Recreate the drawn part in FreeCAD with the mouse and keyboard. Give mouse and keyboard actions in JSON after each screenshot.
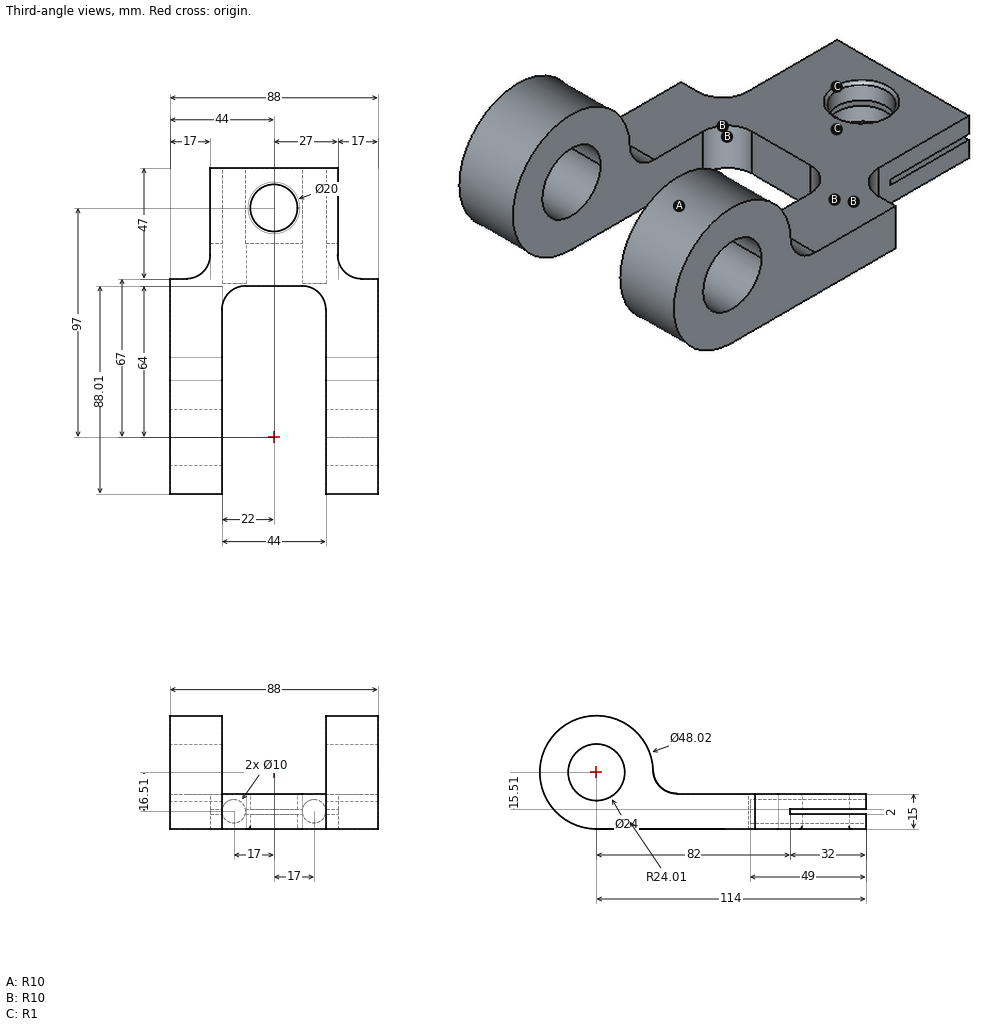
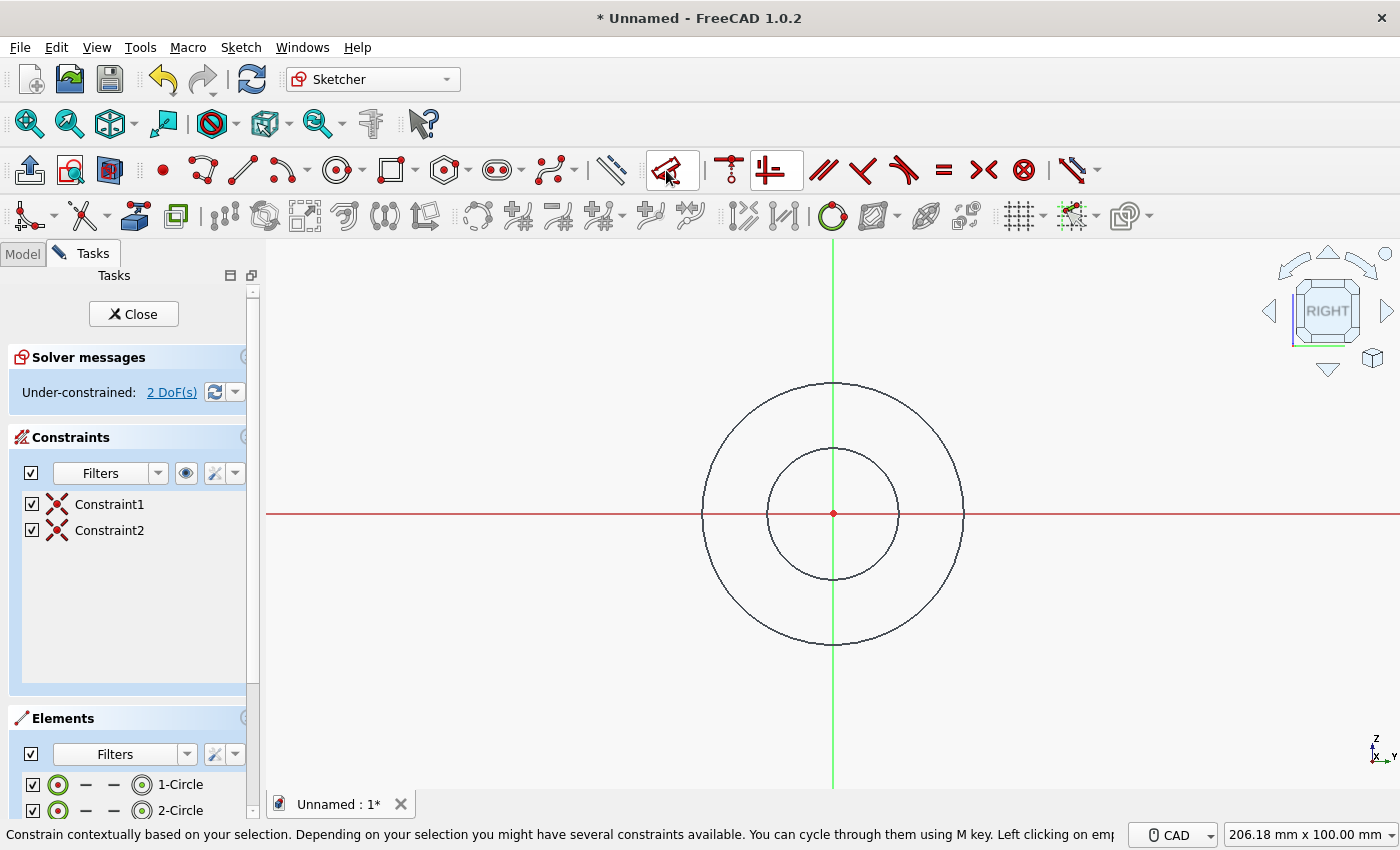
{"action": "left_click", "coordinate": [925, 421]}
{"action": "left_click", "coordinate": [948, 398]}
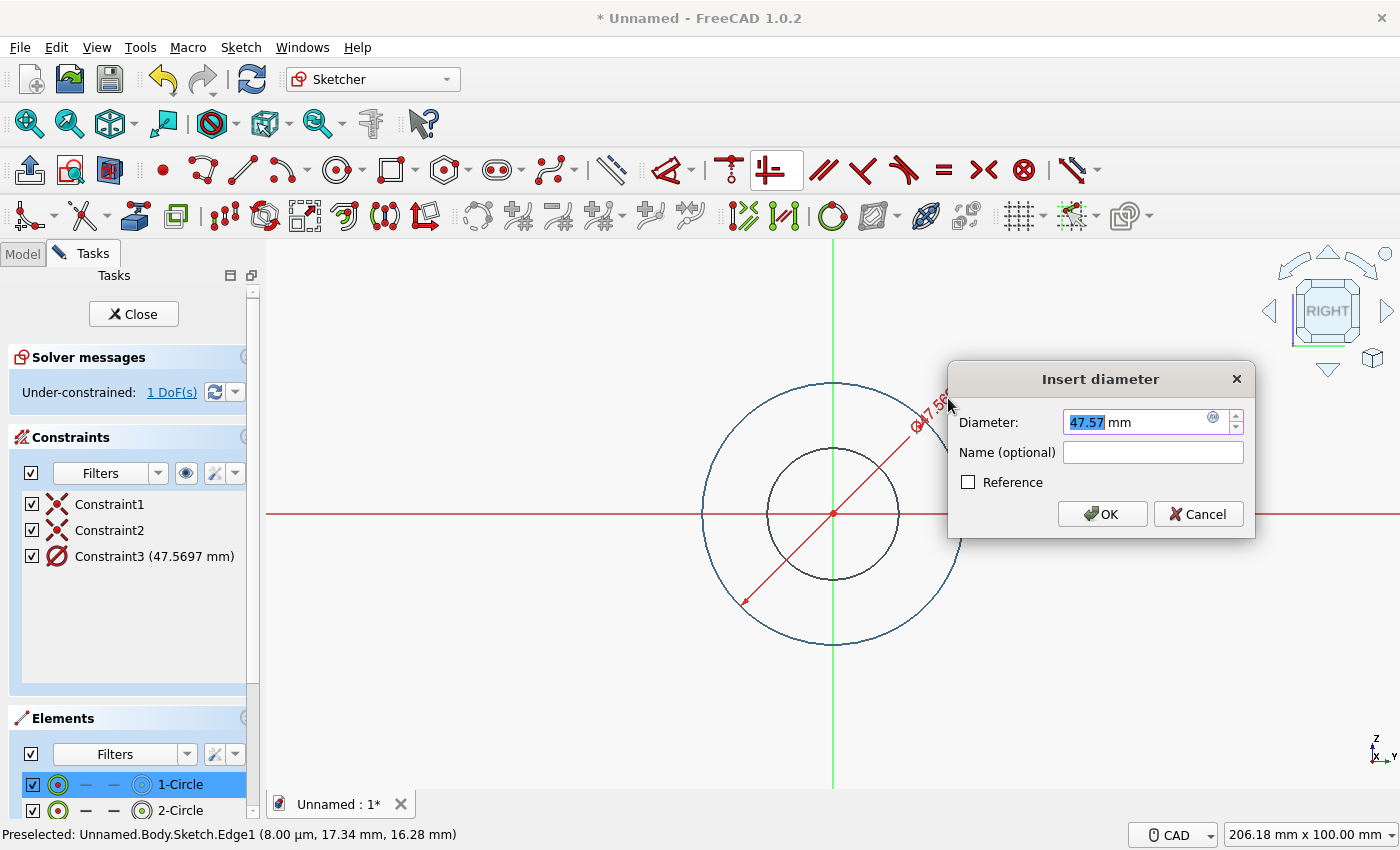
{"action": "type", "text": "48.02"}
{"action": "key", "text": "Return"}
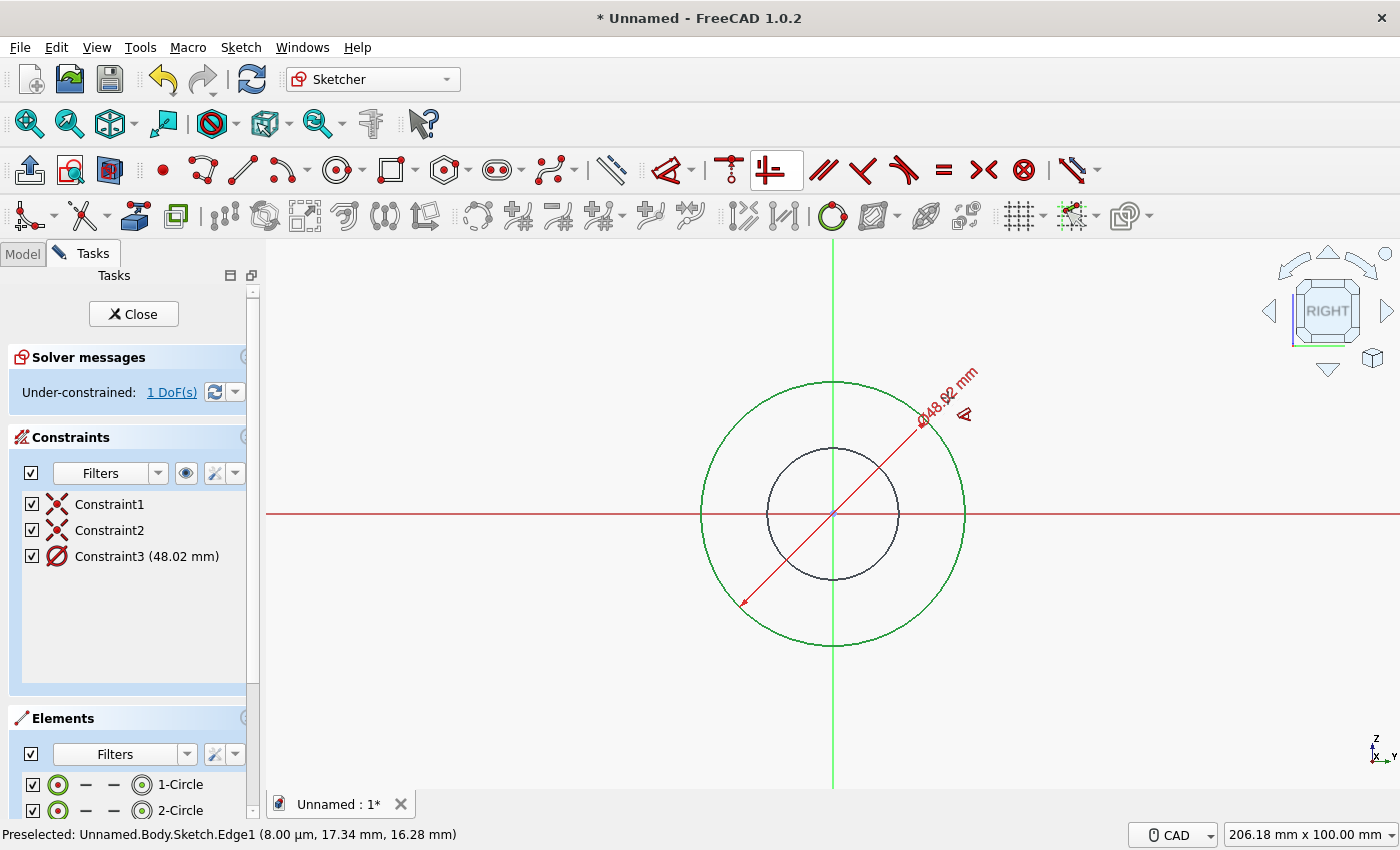
{"action": "left_click", "coordinate": [879, 467]}
{"action": "left_click", "coordinate": [901, 444]}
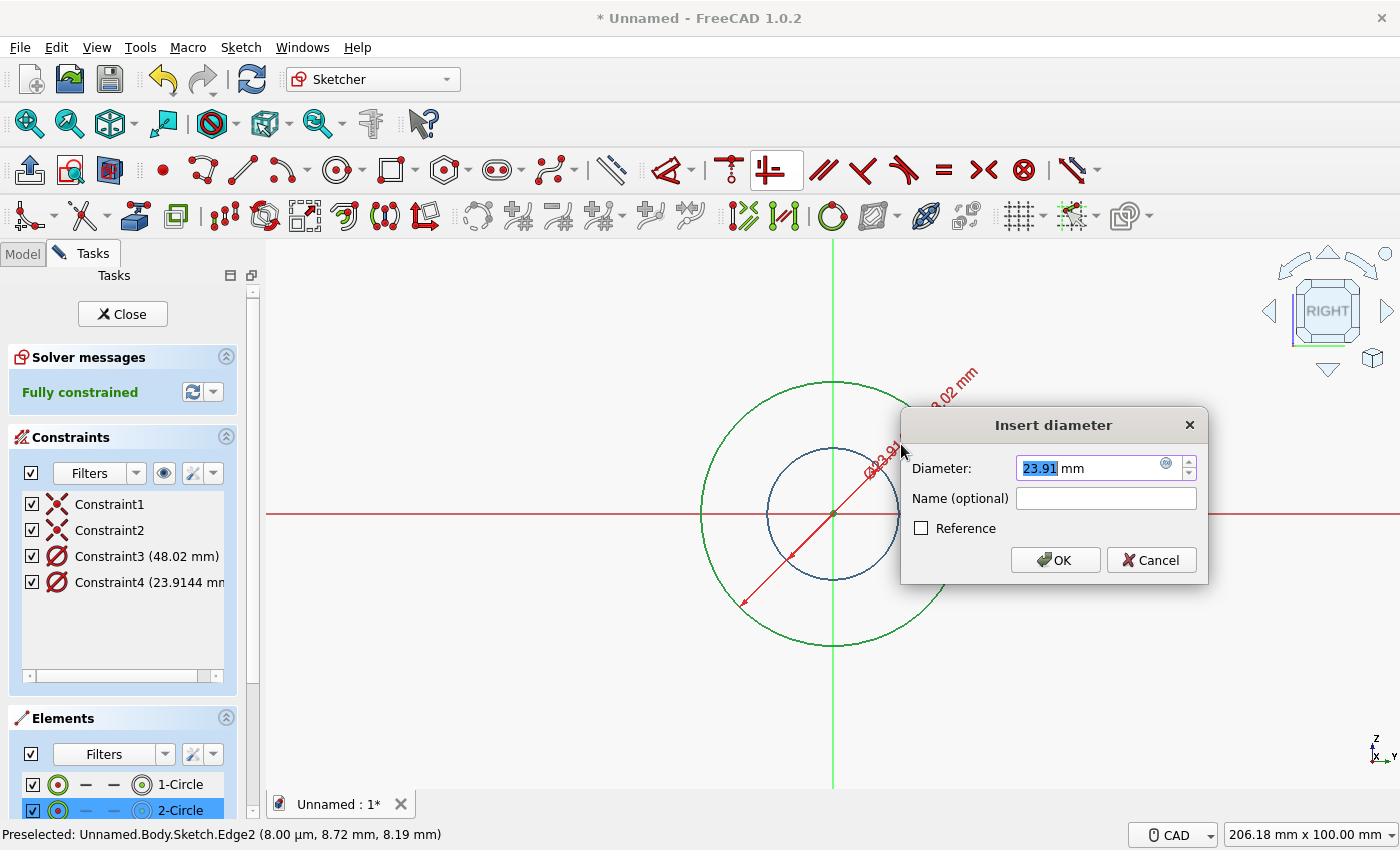
{"action": "type", "text": "24"}
{"action": "key", "text": "Return"}
{"action": "key", "text": "Escape"}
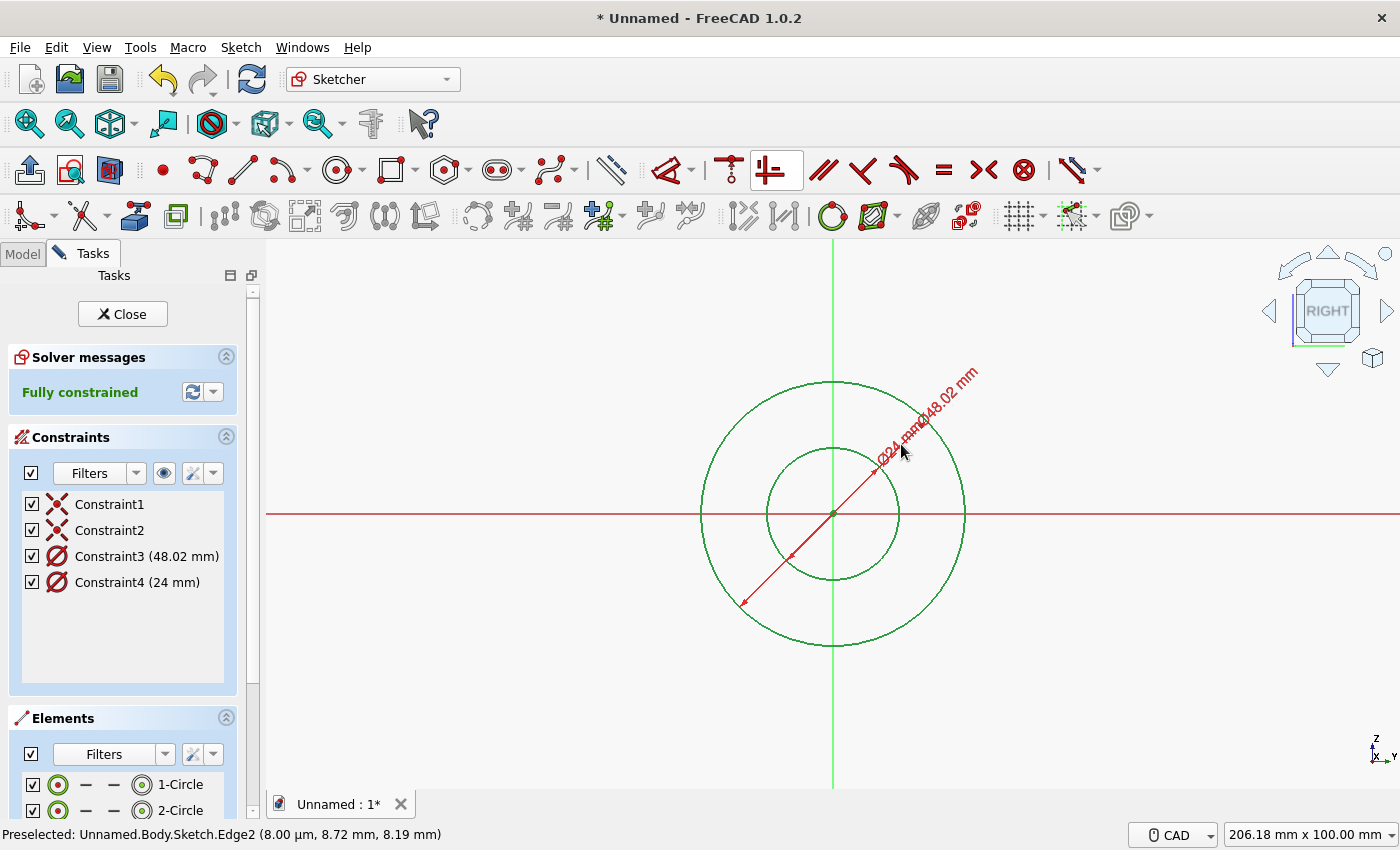
{"action": "left_click", "coordinate": [123, 314]}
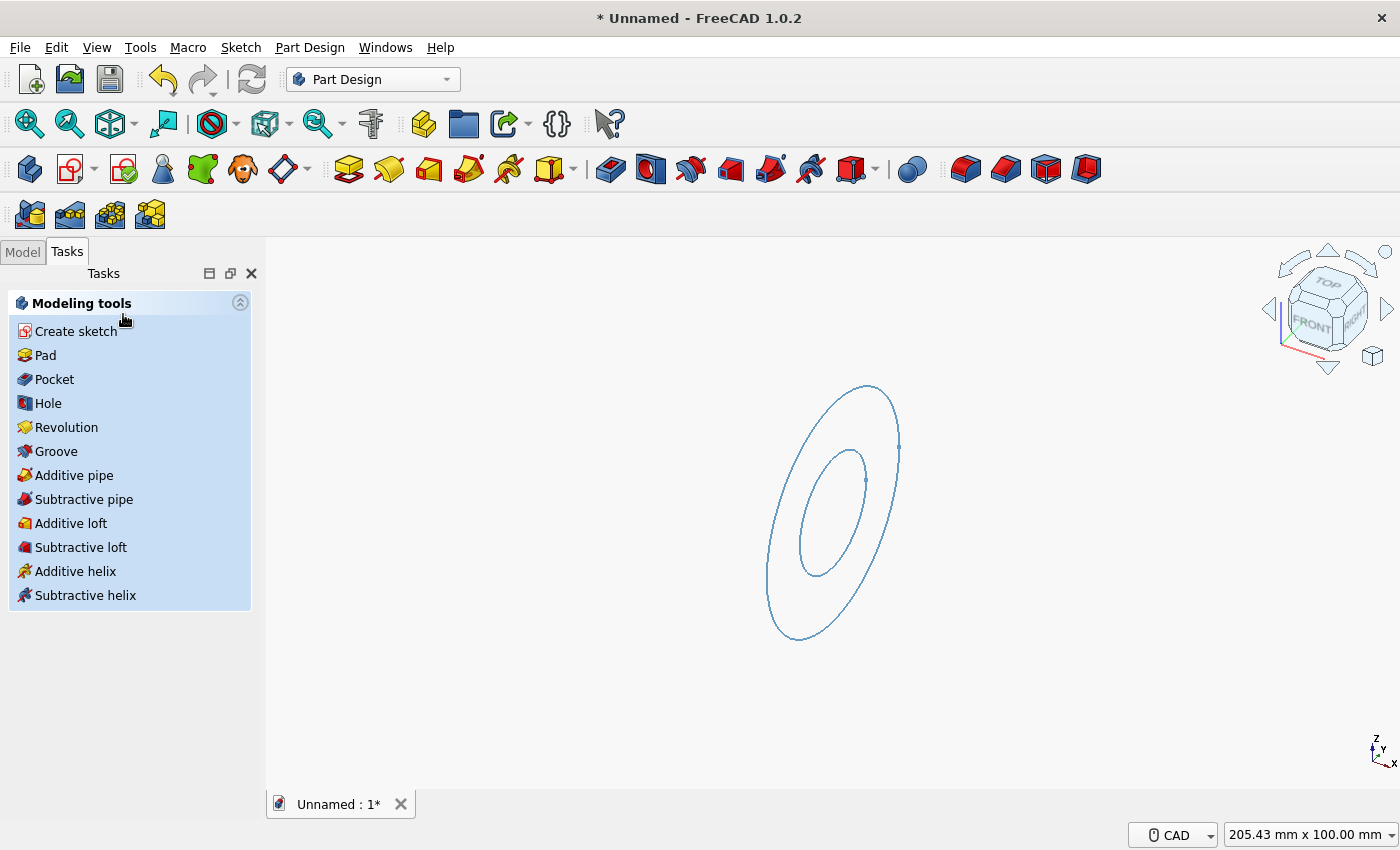
{"action": "left_click", "coordinate": [350, 170]}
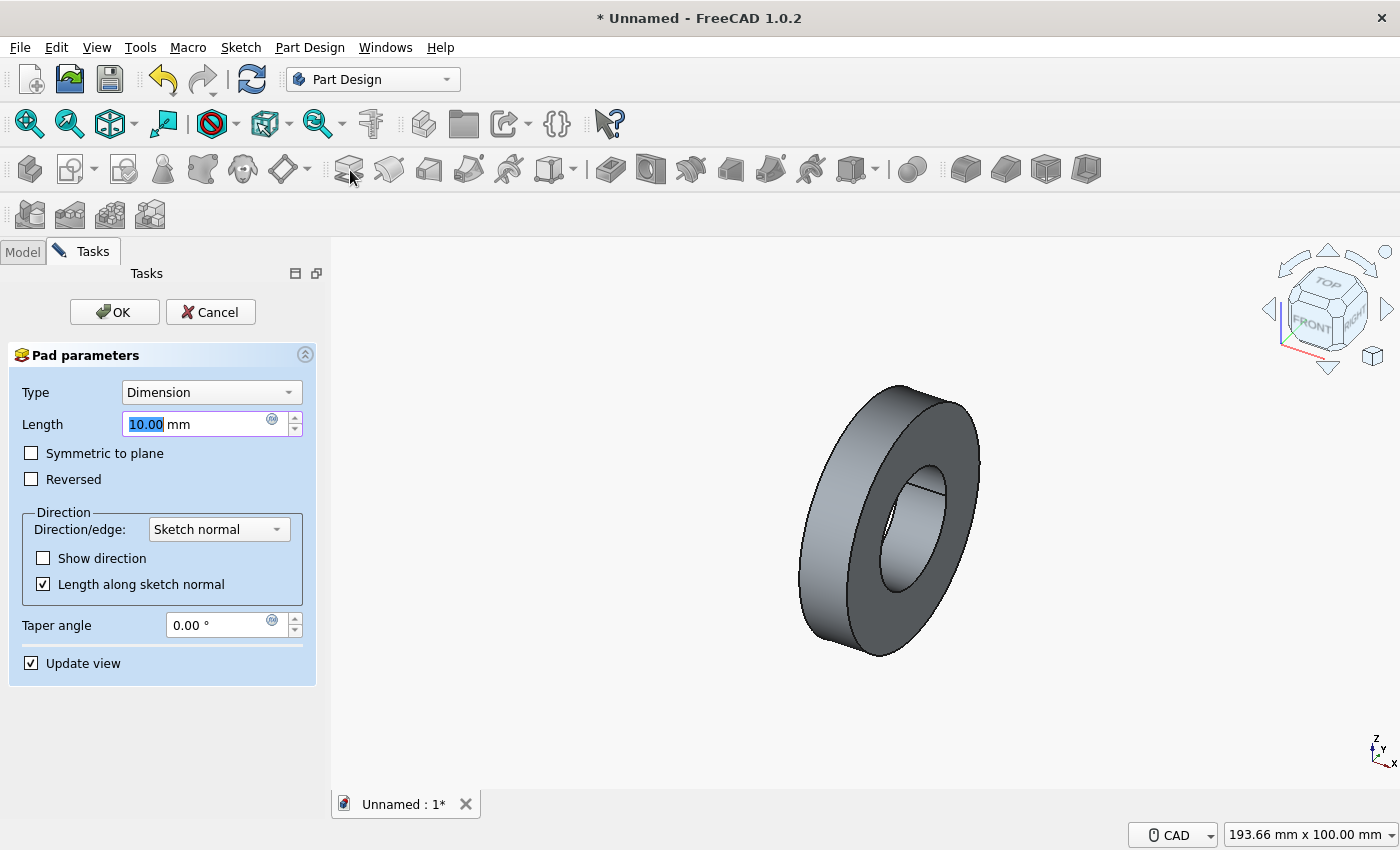
{"action": "type", "text": "88"}
{"action": "key", "text": "Tab"}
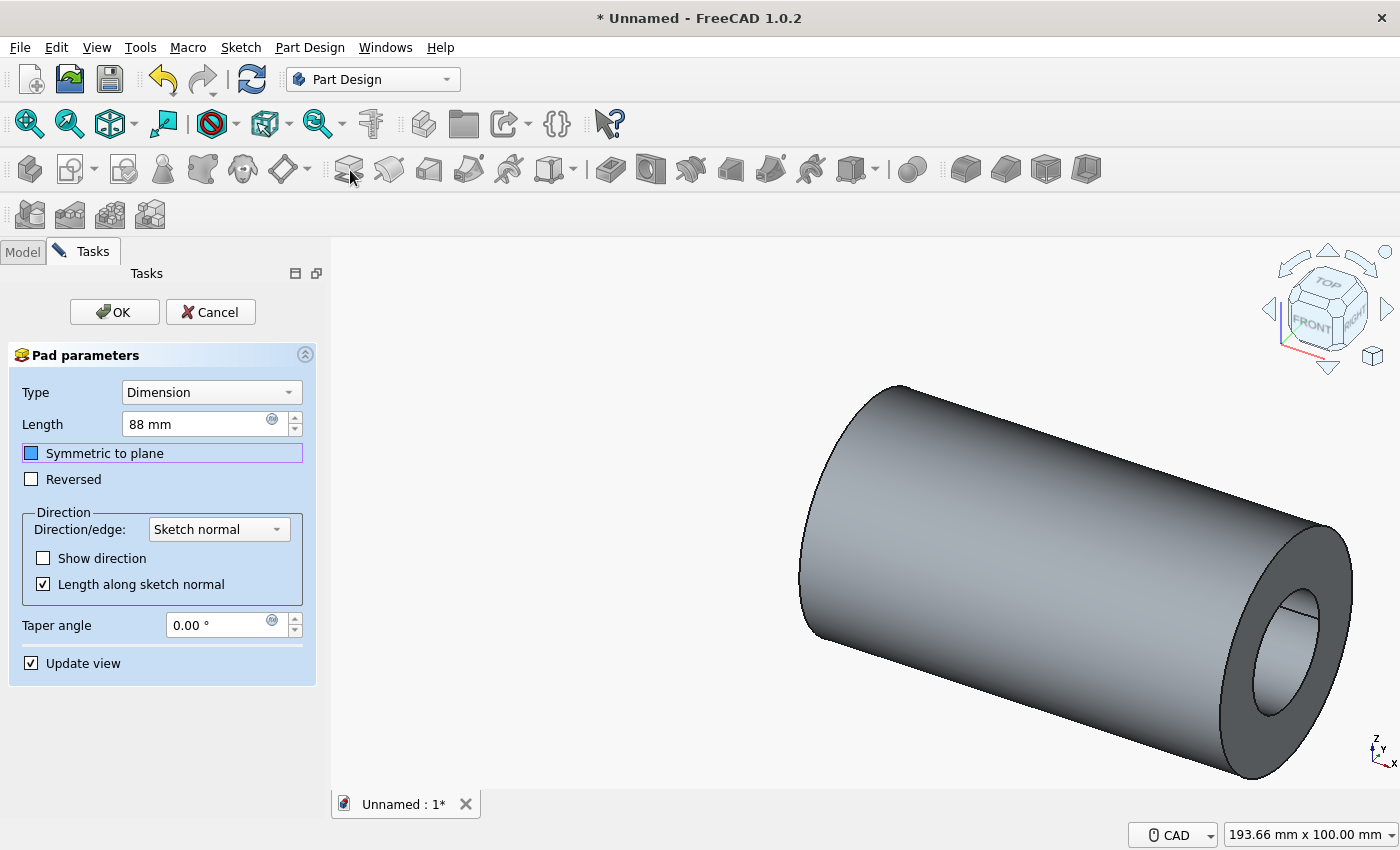
{"action": "left_click", "coordinate": [30, 453]}